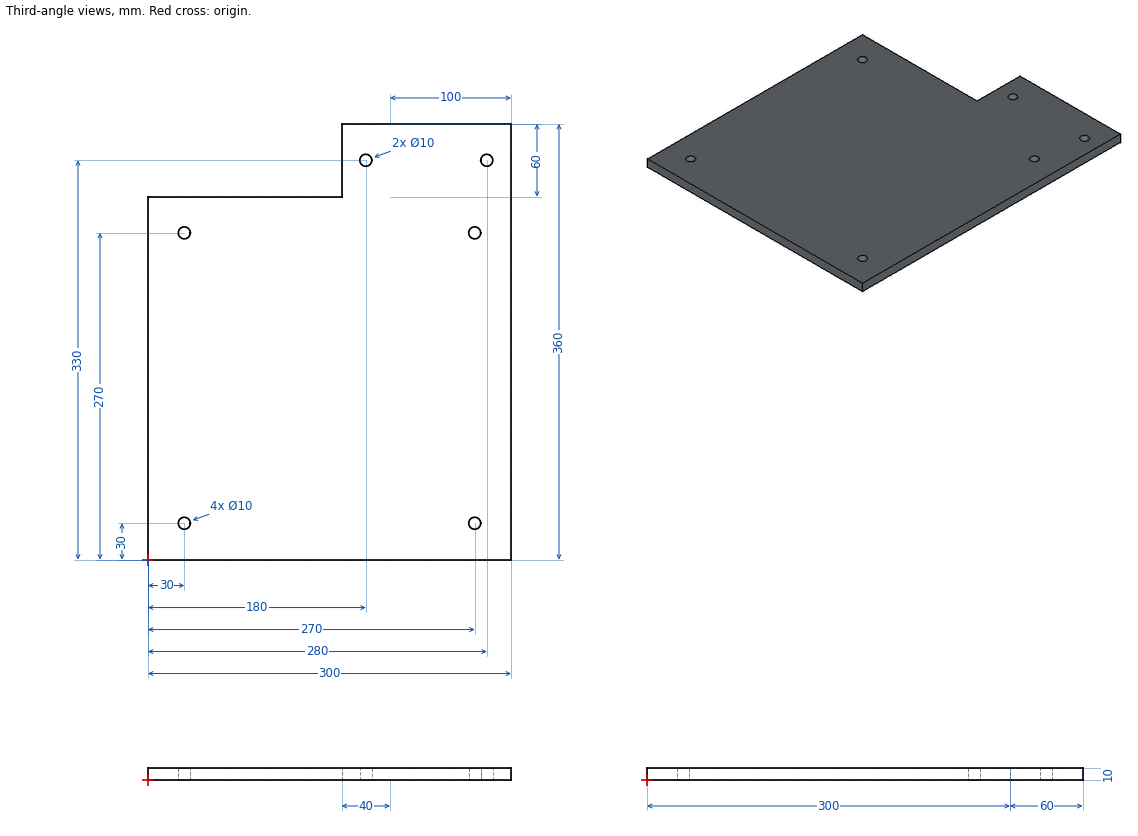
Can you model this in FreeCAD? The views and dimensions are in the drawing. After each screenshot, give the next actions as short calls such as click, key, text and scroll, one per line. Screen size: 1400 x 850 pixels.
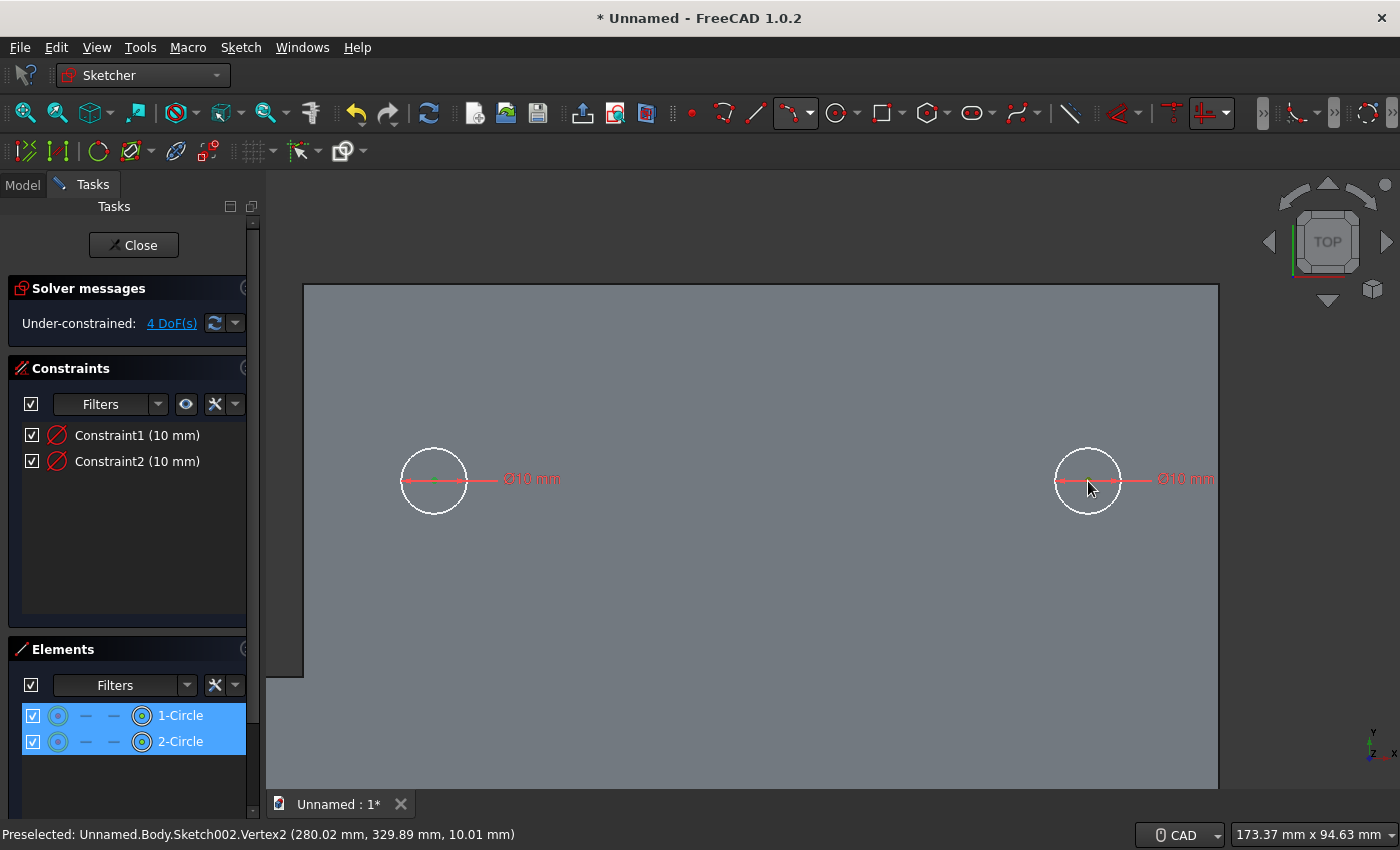
click(1228, 114)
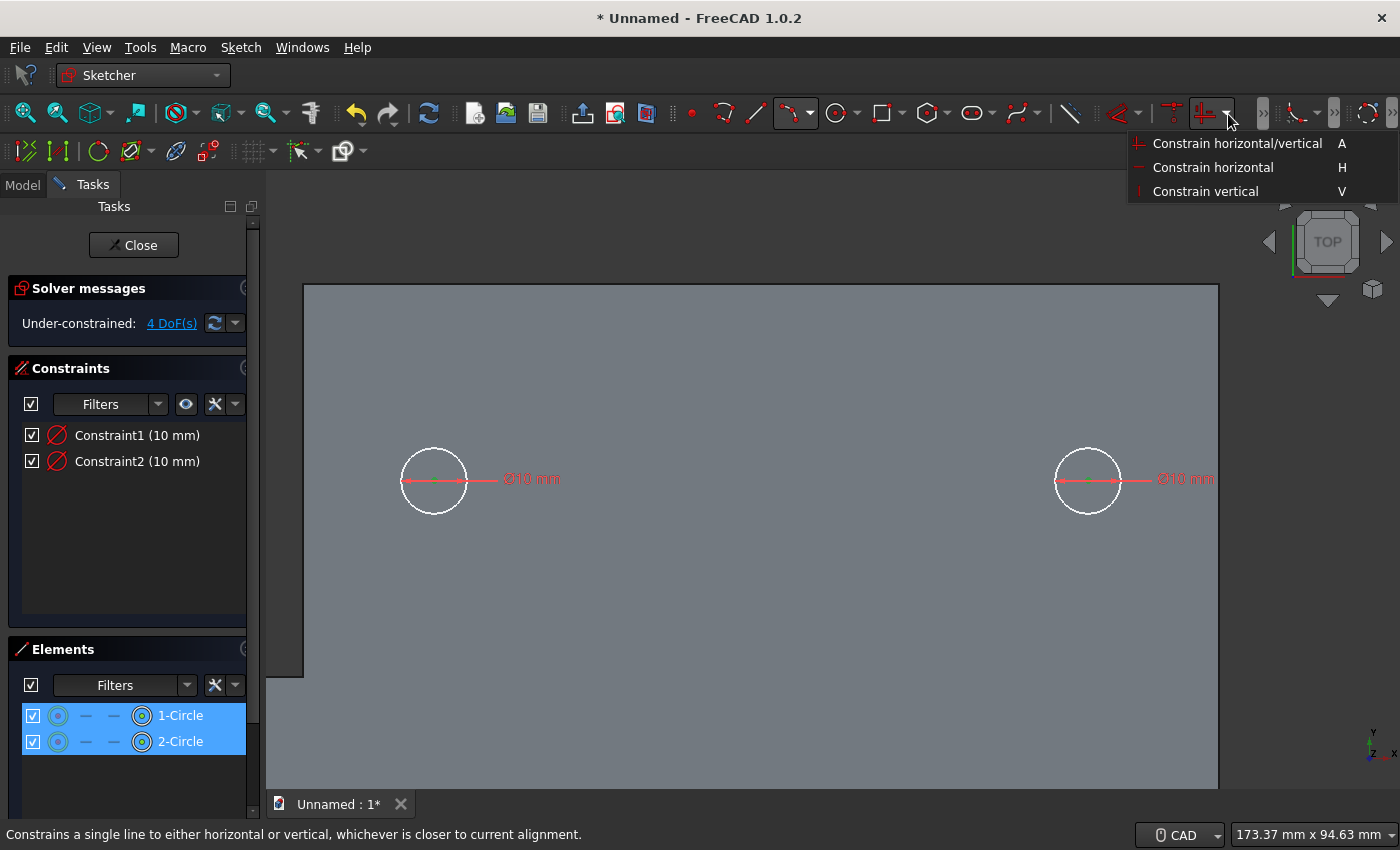
click(1263, 167)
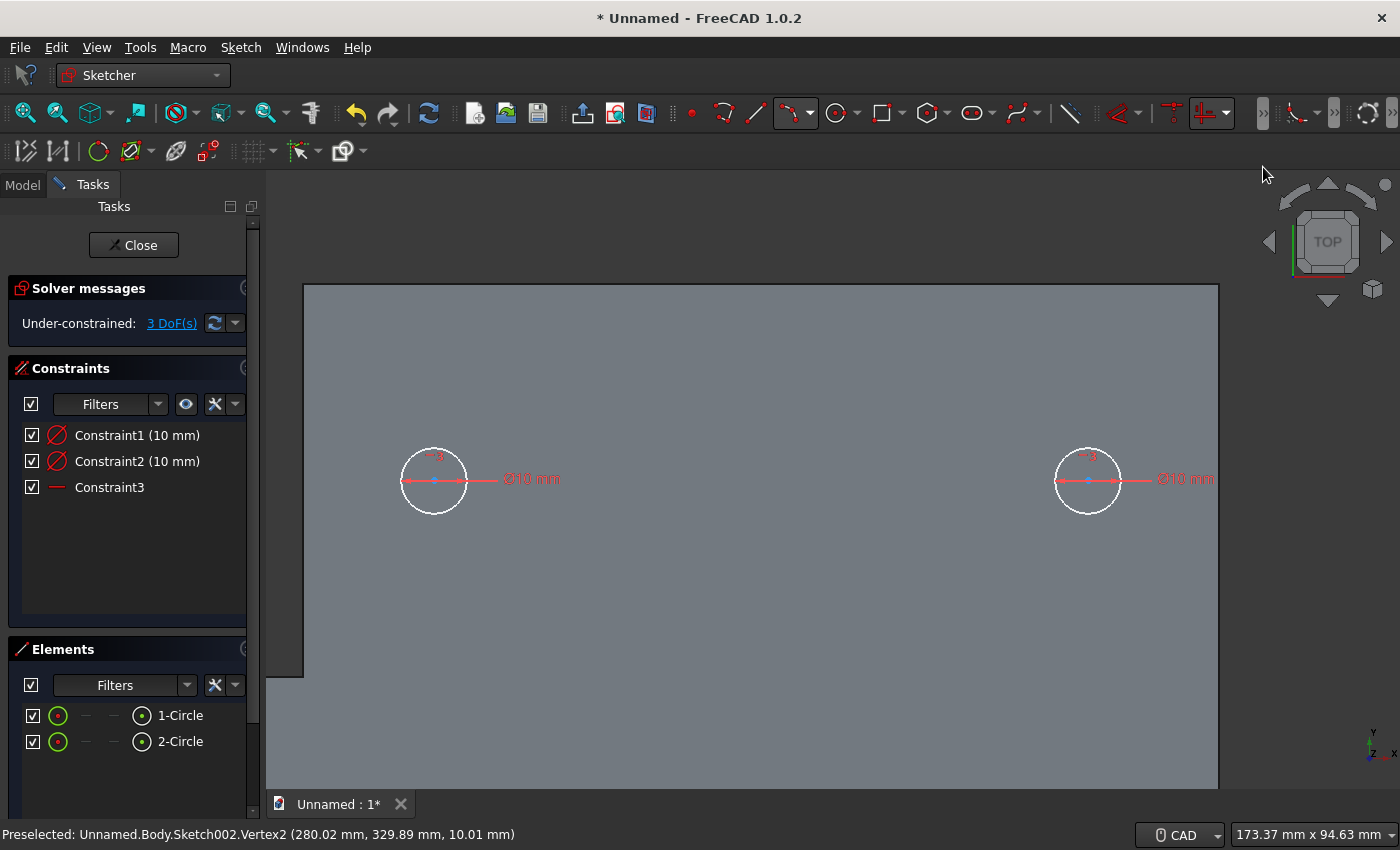
click(1118, 114)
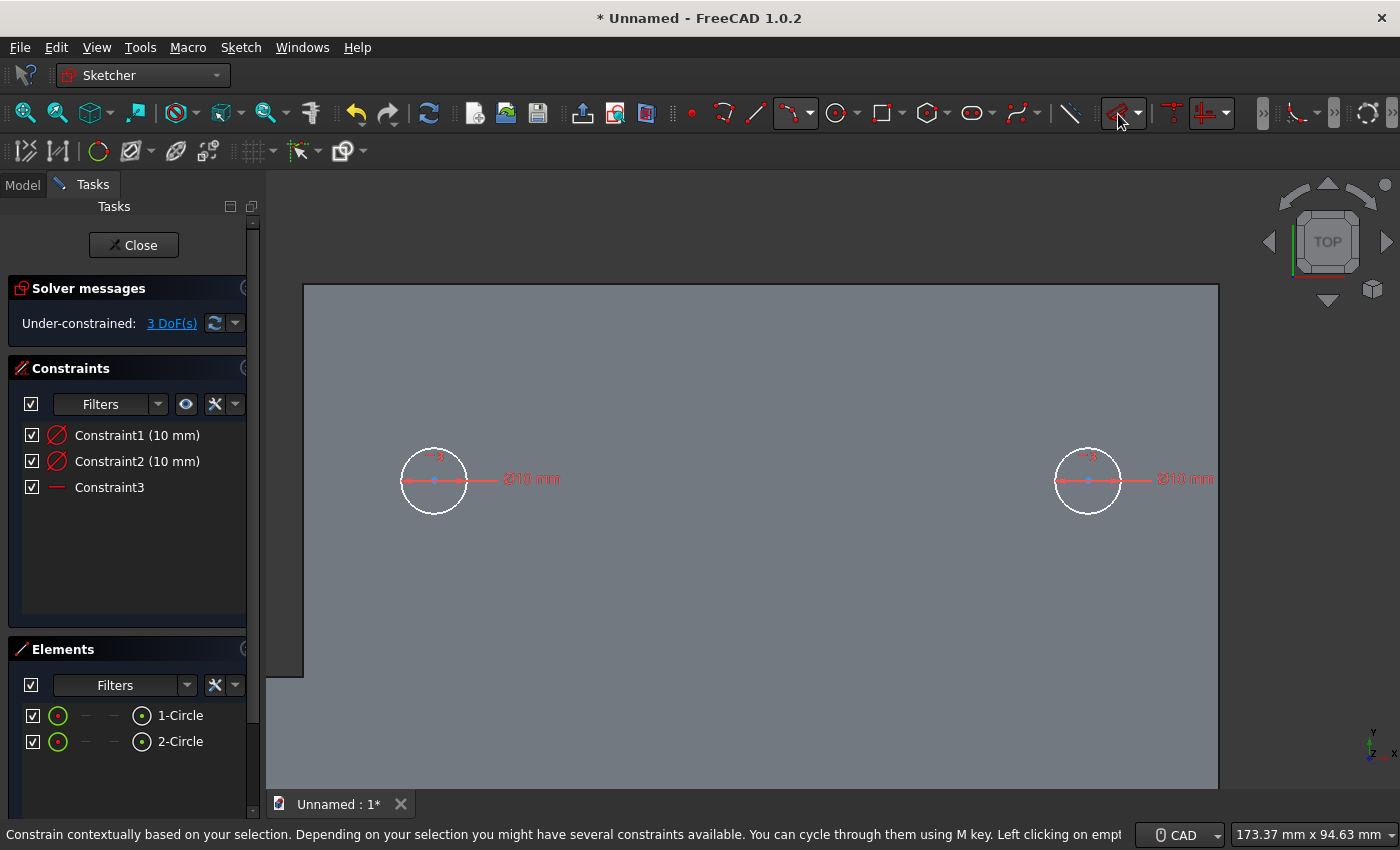
click(434, 481)
click(364, 447)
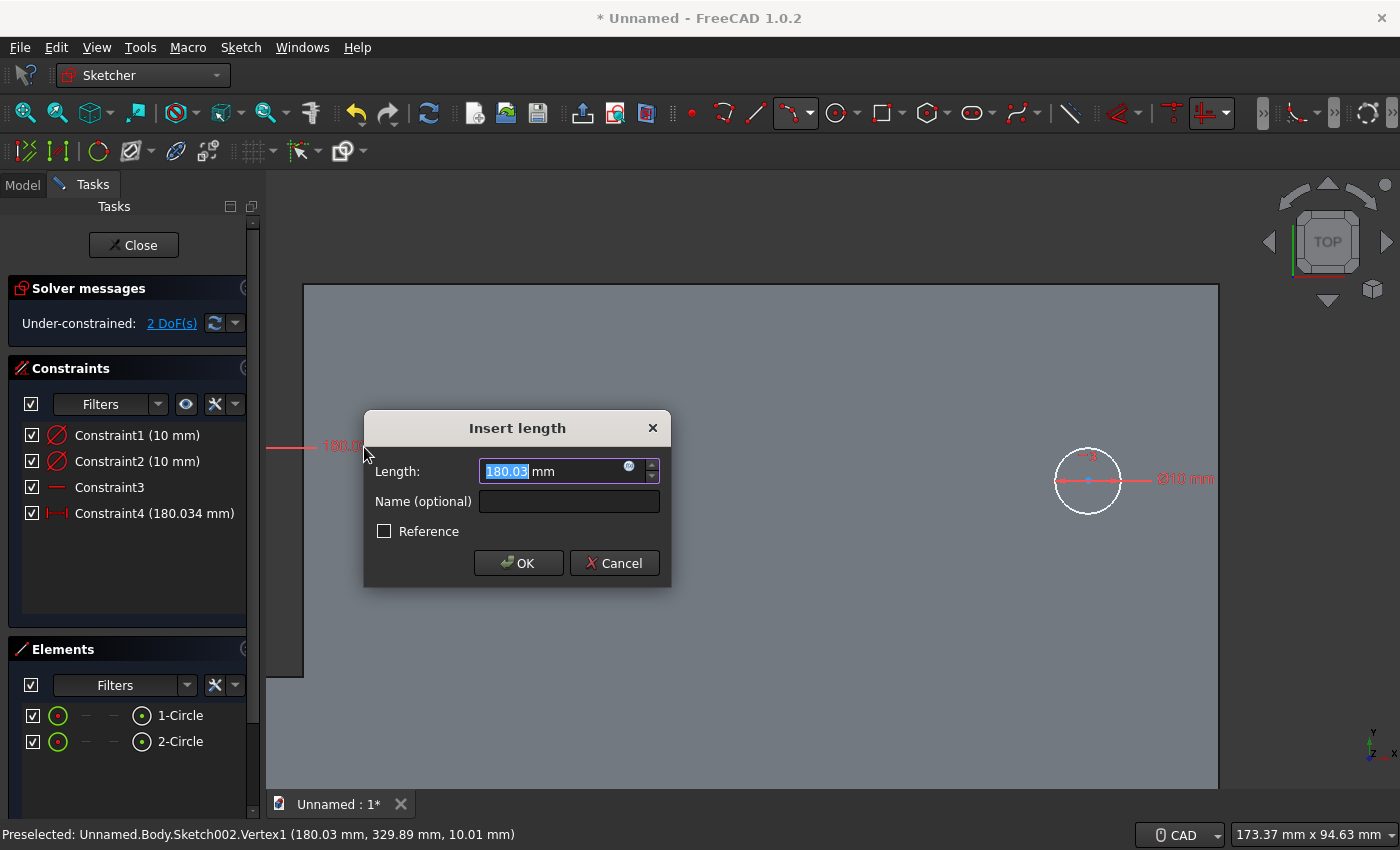
text(180)
key(Return)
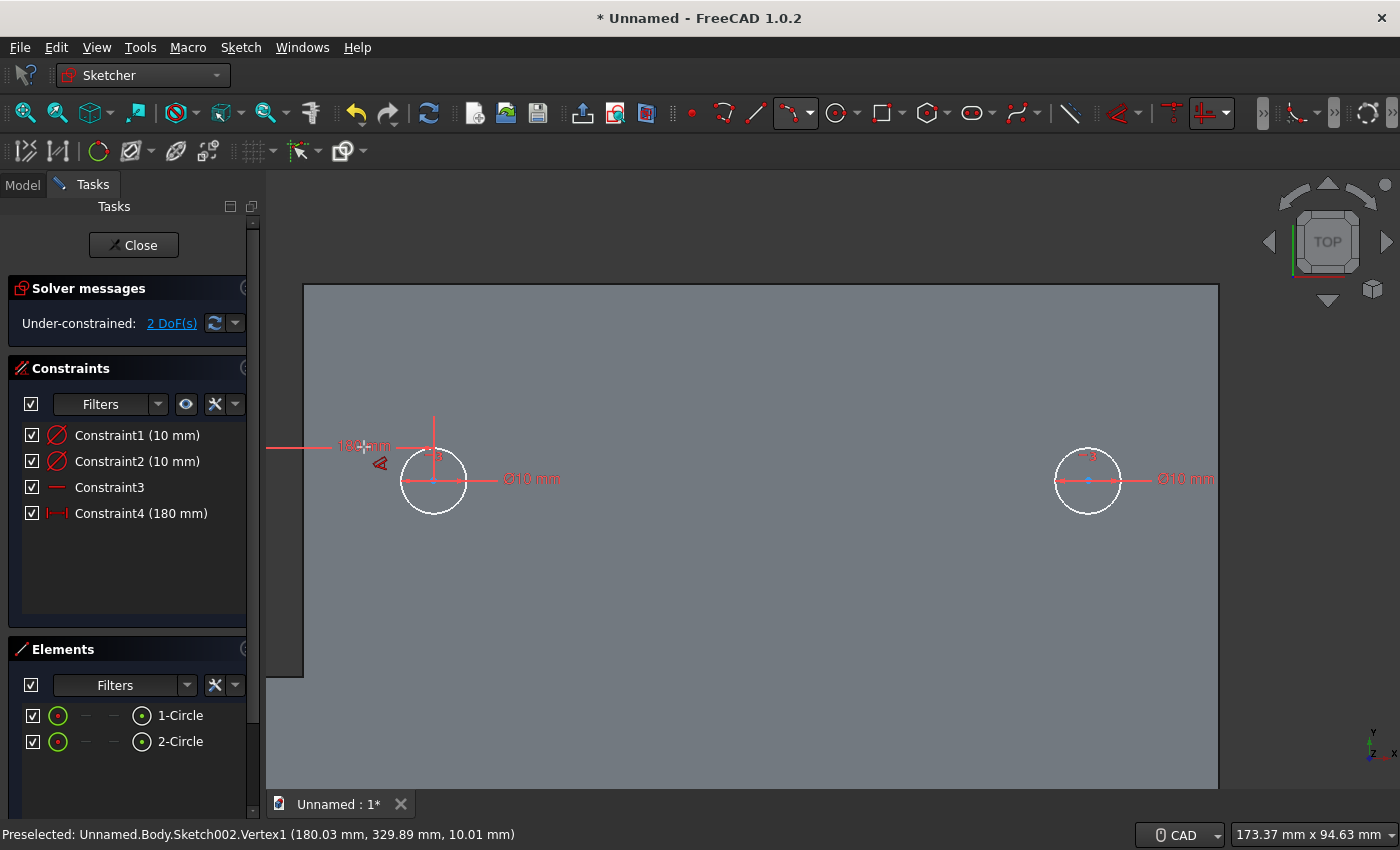
click(434, 481)
click(468, 621)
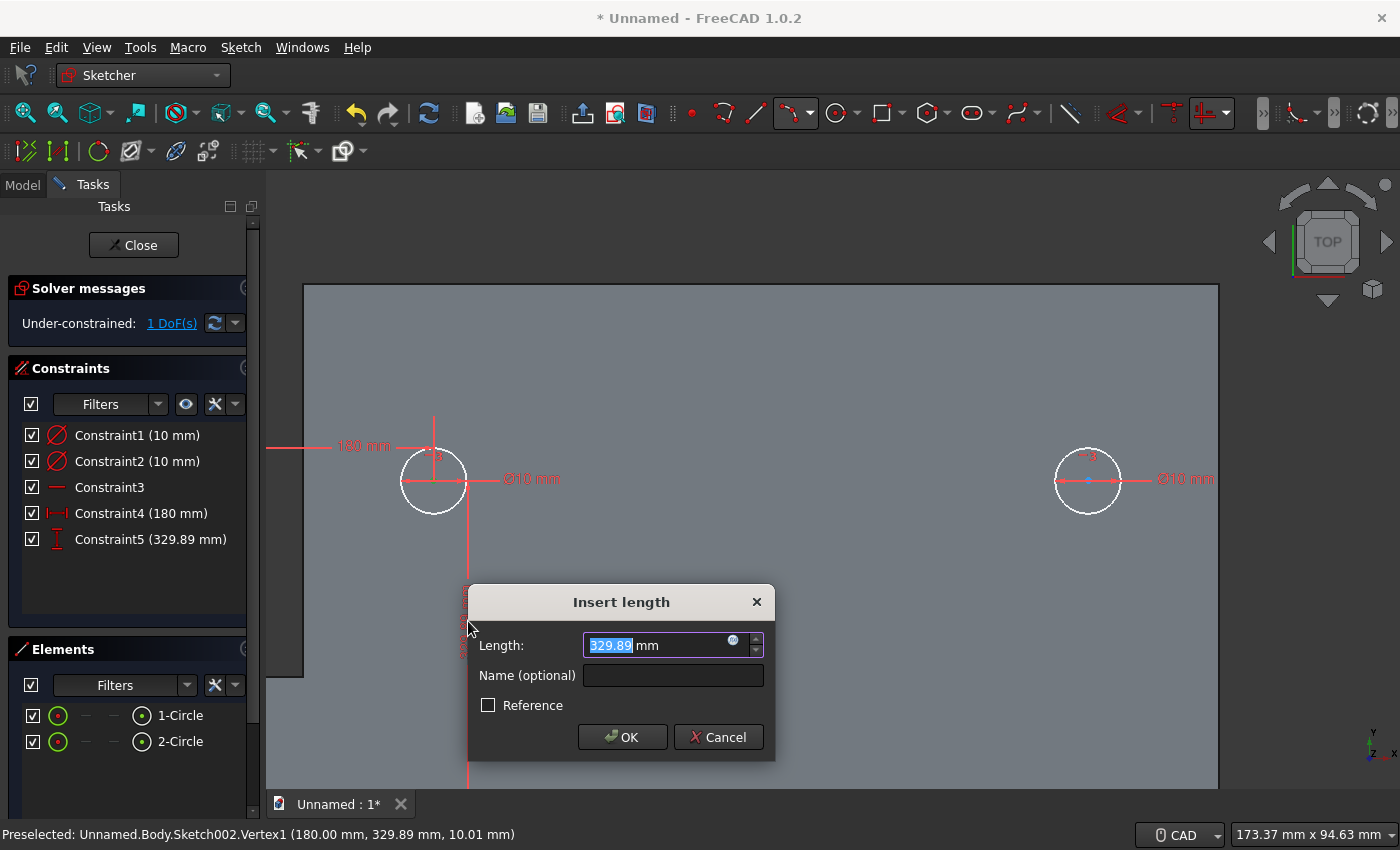
text(330)
key(Return)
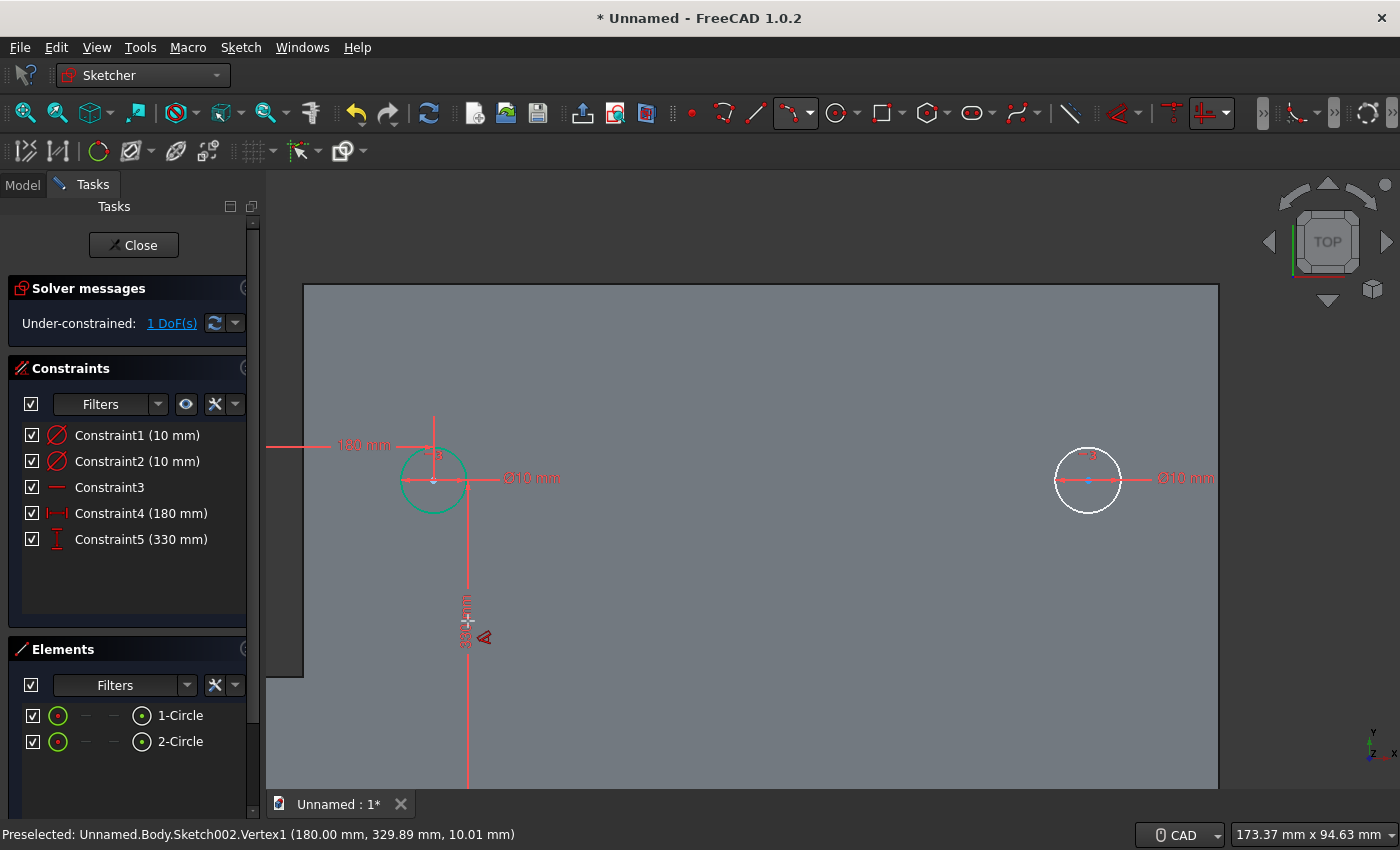
click(1088, 480)
click(691, 446)